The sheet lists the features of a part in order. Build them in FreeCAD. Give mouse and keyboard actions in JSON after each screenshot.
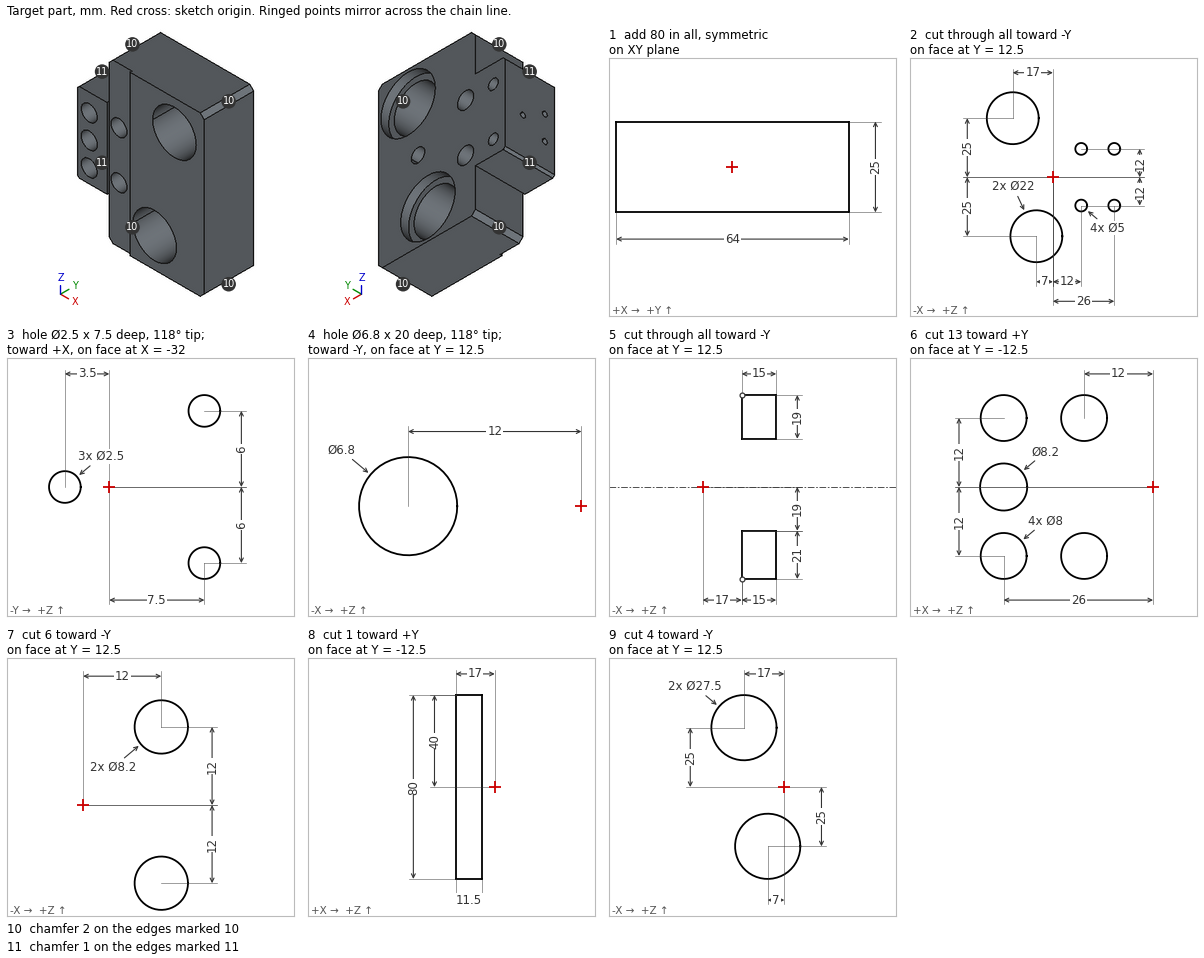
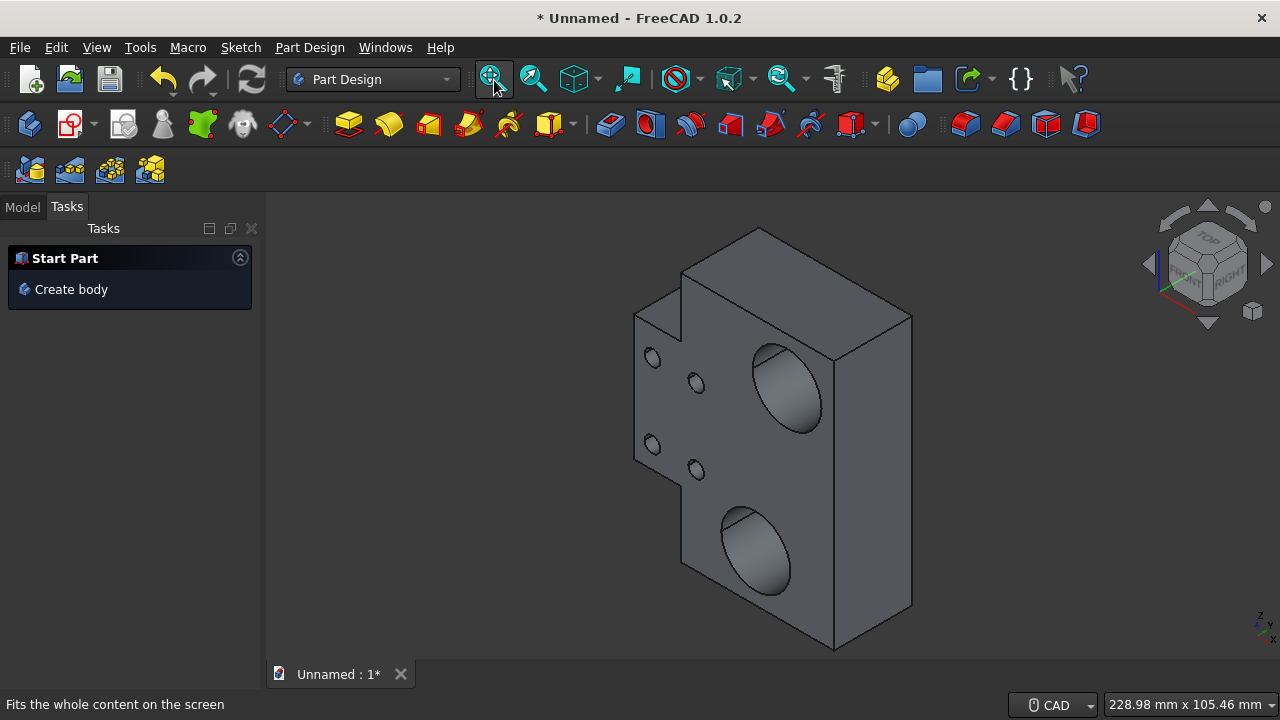
{"action": "left_click", "coordinate": [734, 447]}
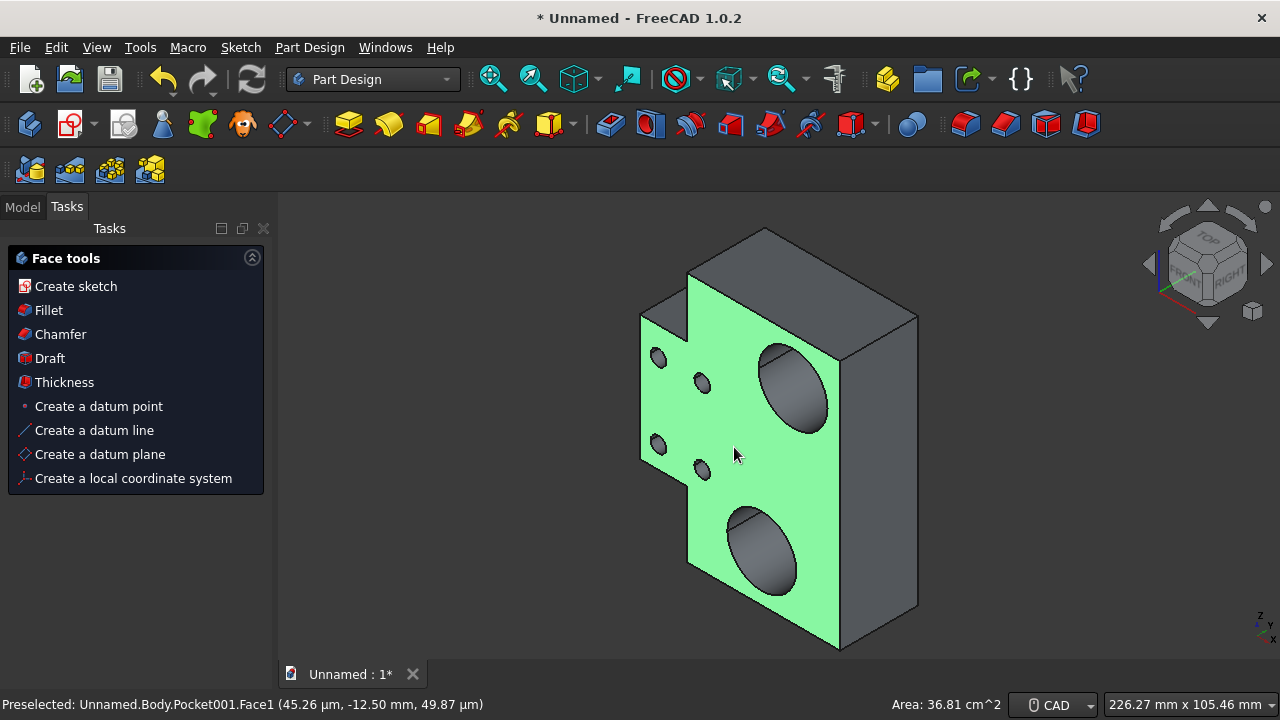
{"action": "left_click", "coordinate": [70, 124]}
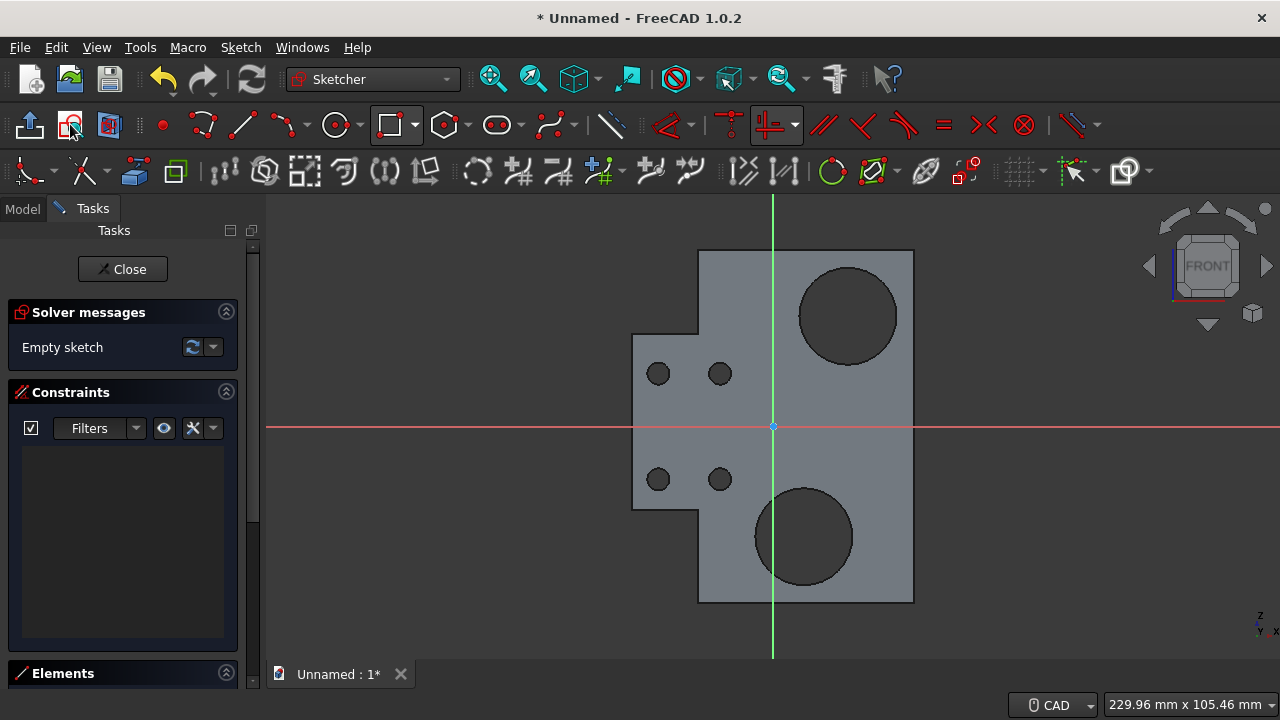
{"action": "scroll", "coordinate": [708, 426], "scroll_direction": "up", "scroll_amount": 4}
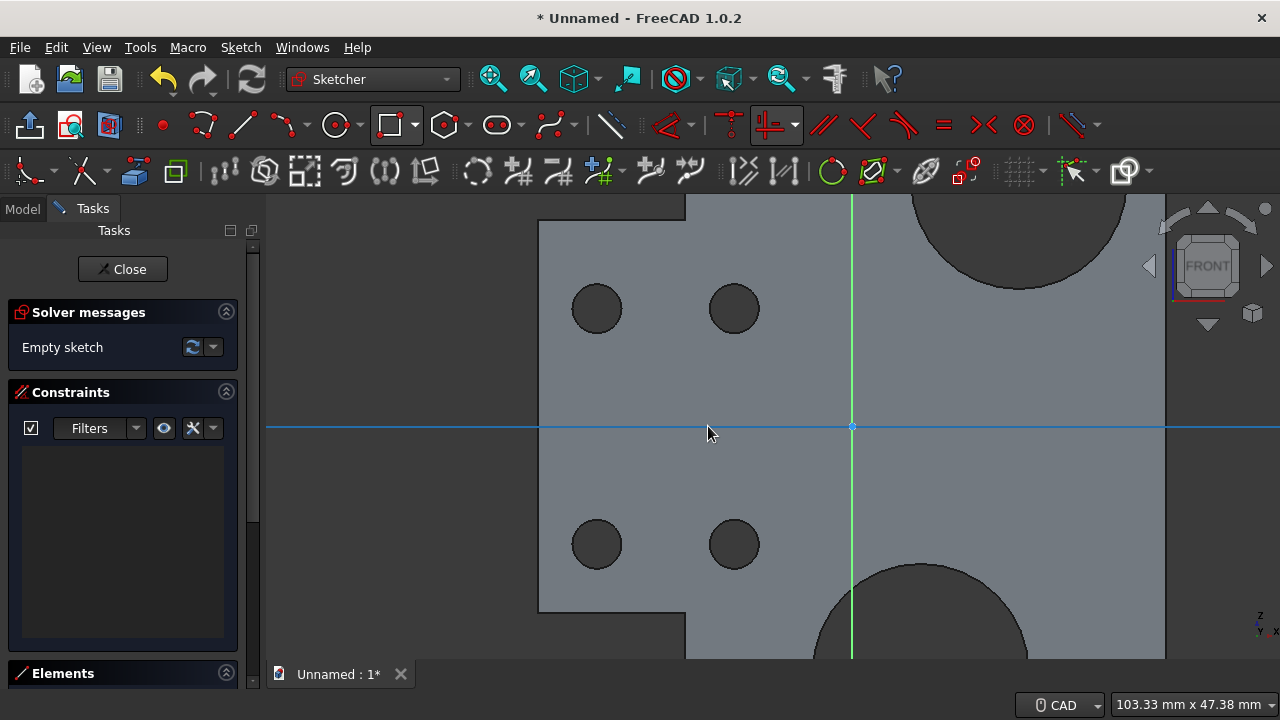
{"action": "left_click", "coordinate": [336, 126]}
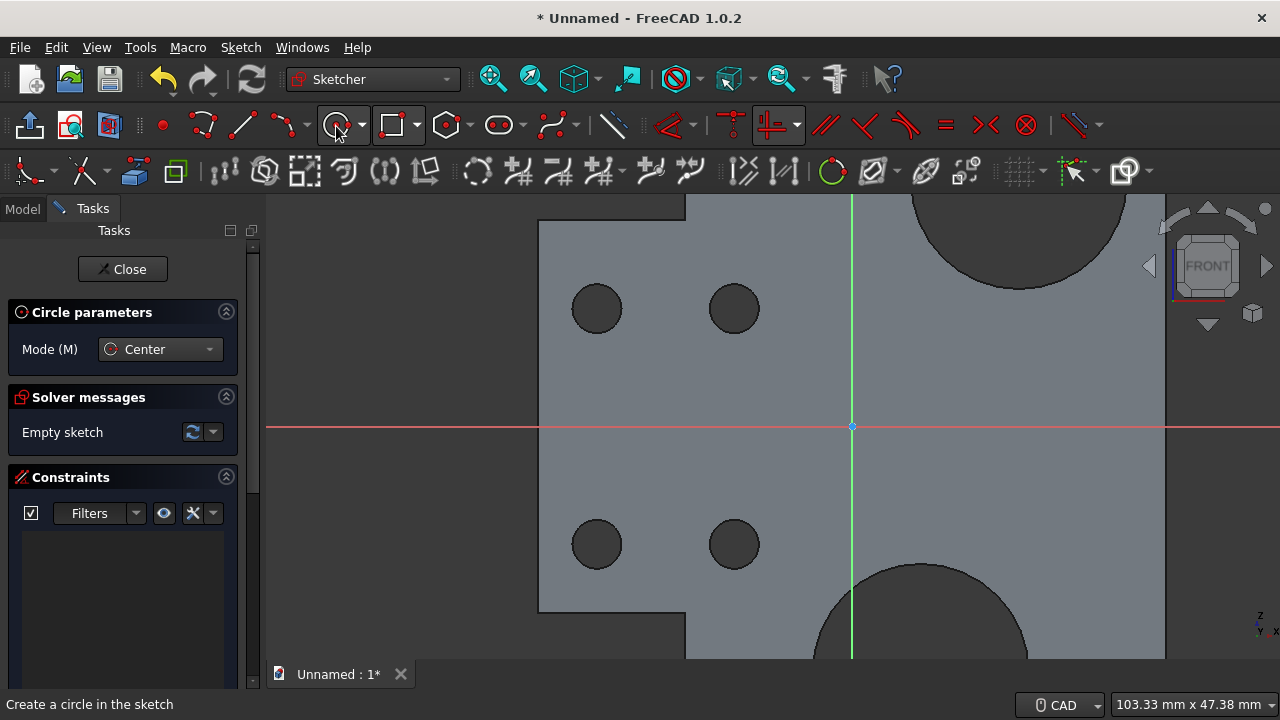
{"action": "left_click", "coordinate": [597, 544]}
{"action": "left_click", "coordinate": [625, 517]}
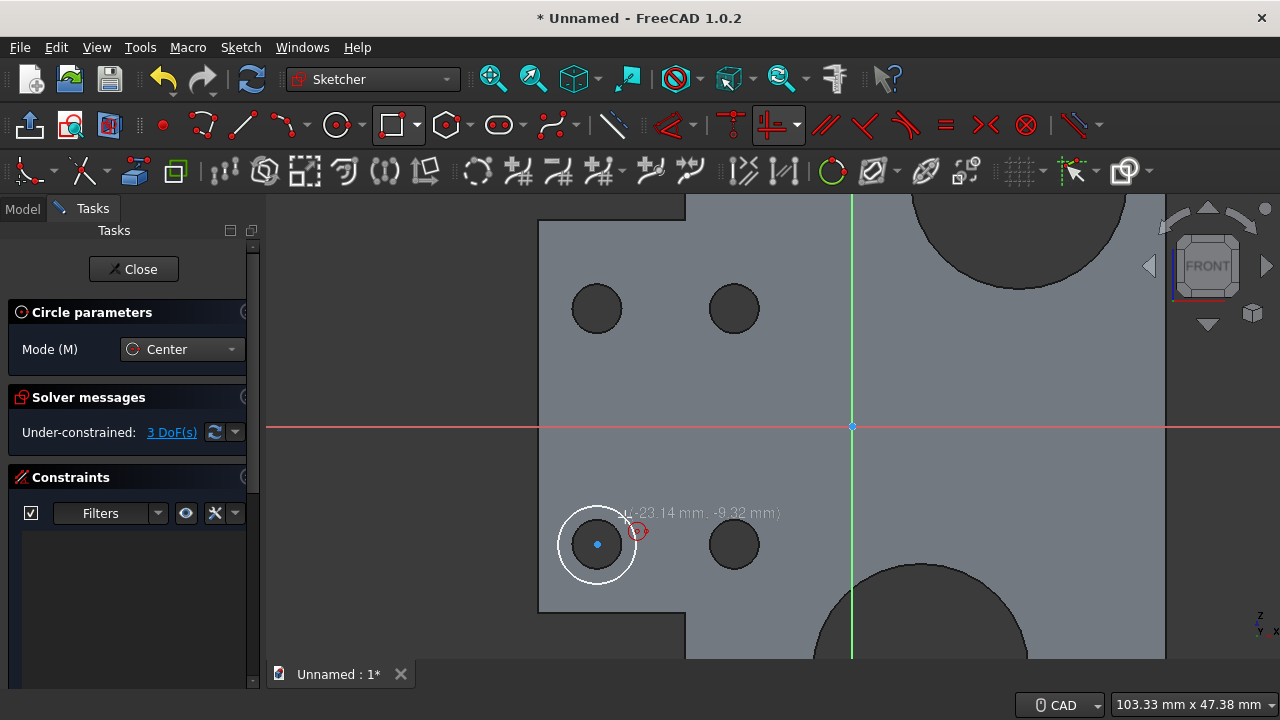
{"action": "left_click", "coordinate": [597, 309]}
{"action": "left_click", "coordinate": [625, 281]}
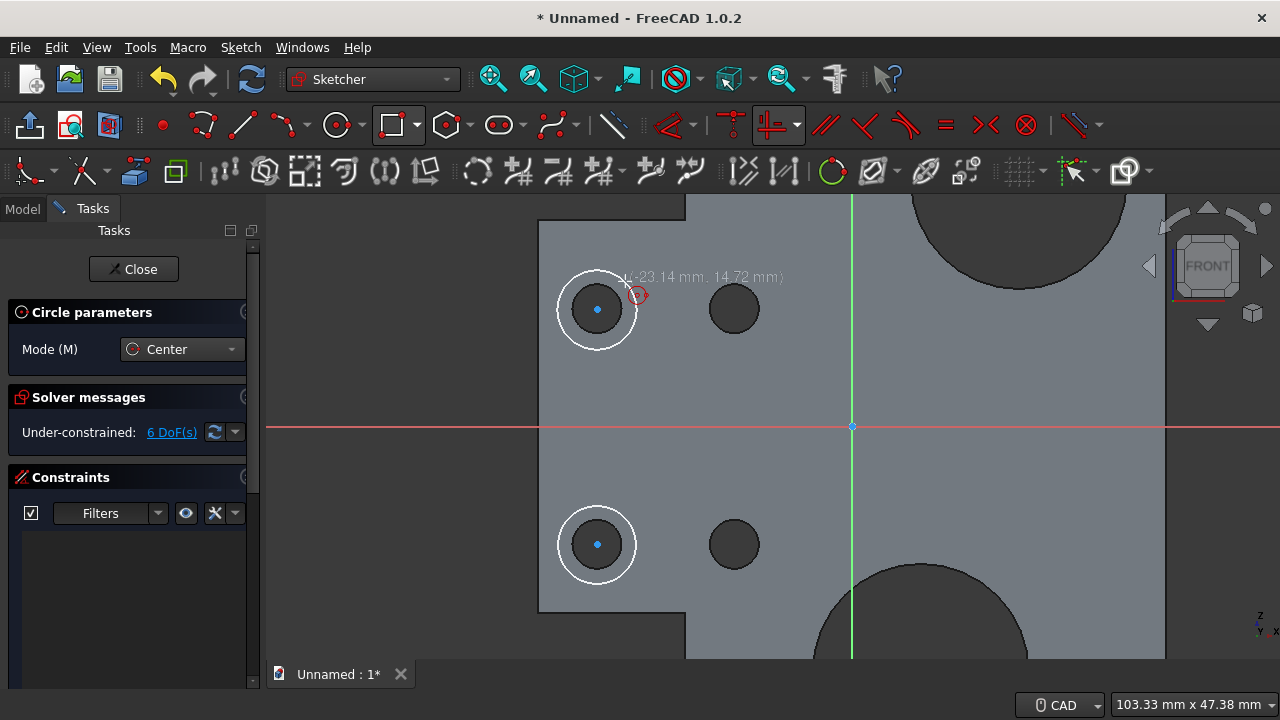
{"action": "left_click", "coordinate": [734, 309]}
{"action": "left_click", "coordinate": [762, 281]}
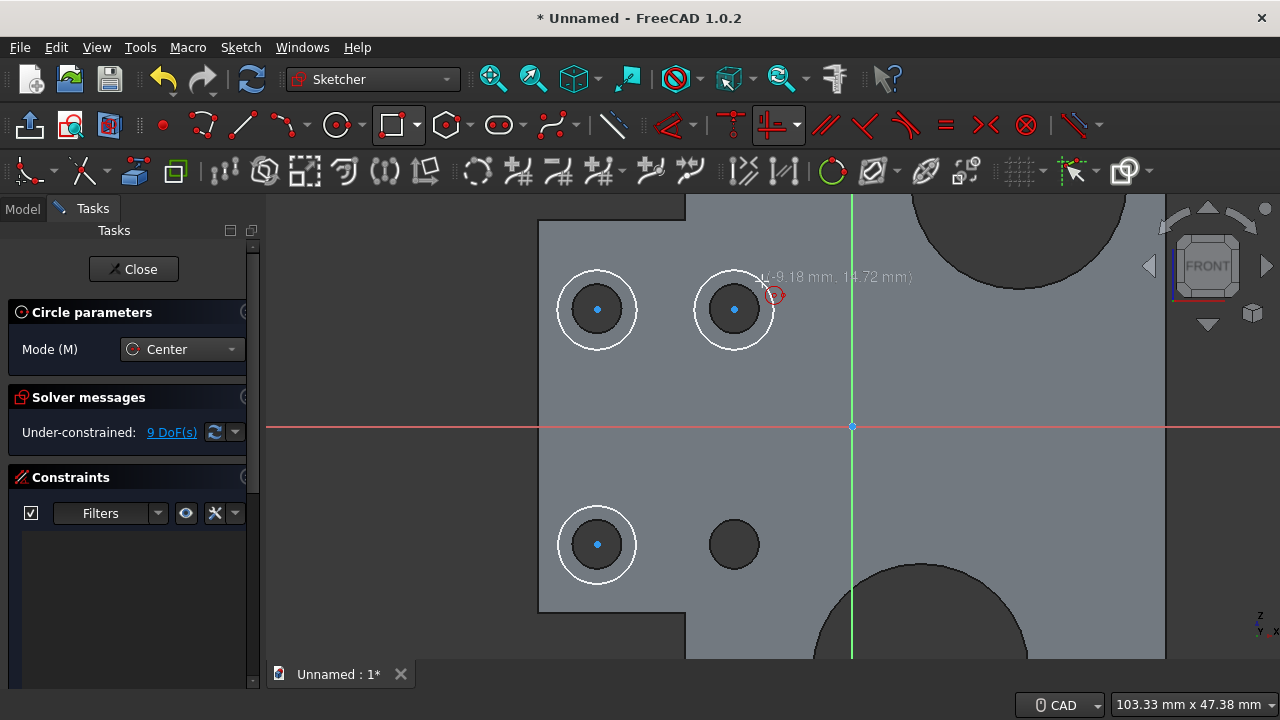
{"action": "left_click", "coordinate": [734, 544]}
{"action": "left_click", "coordinate": [762, 517]}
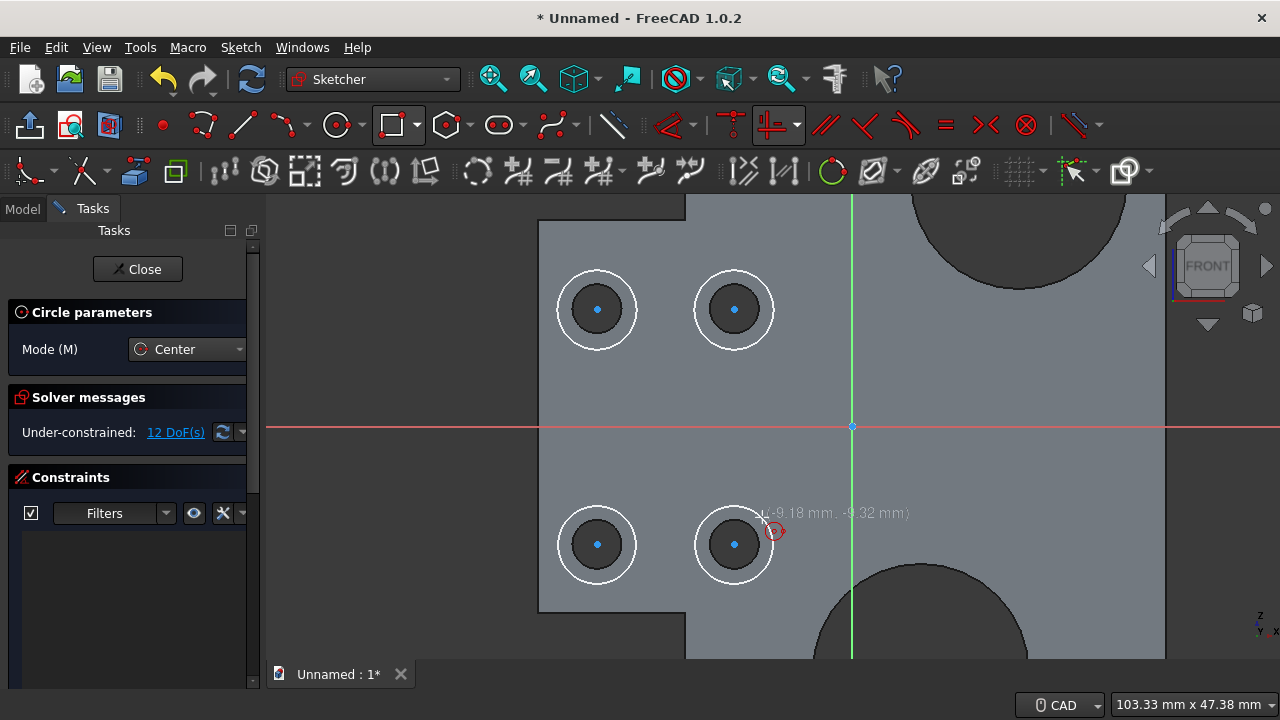
{"action": "left_click", "coordinate": [597, 426]}
{"action": "left_click", "coordinate": [625, 398]}
{"action": "key", "text": "Escape"}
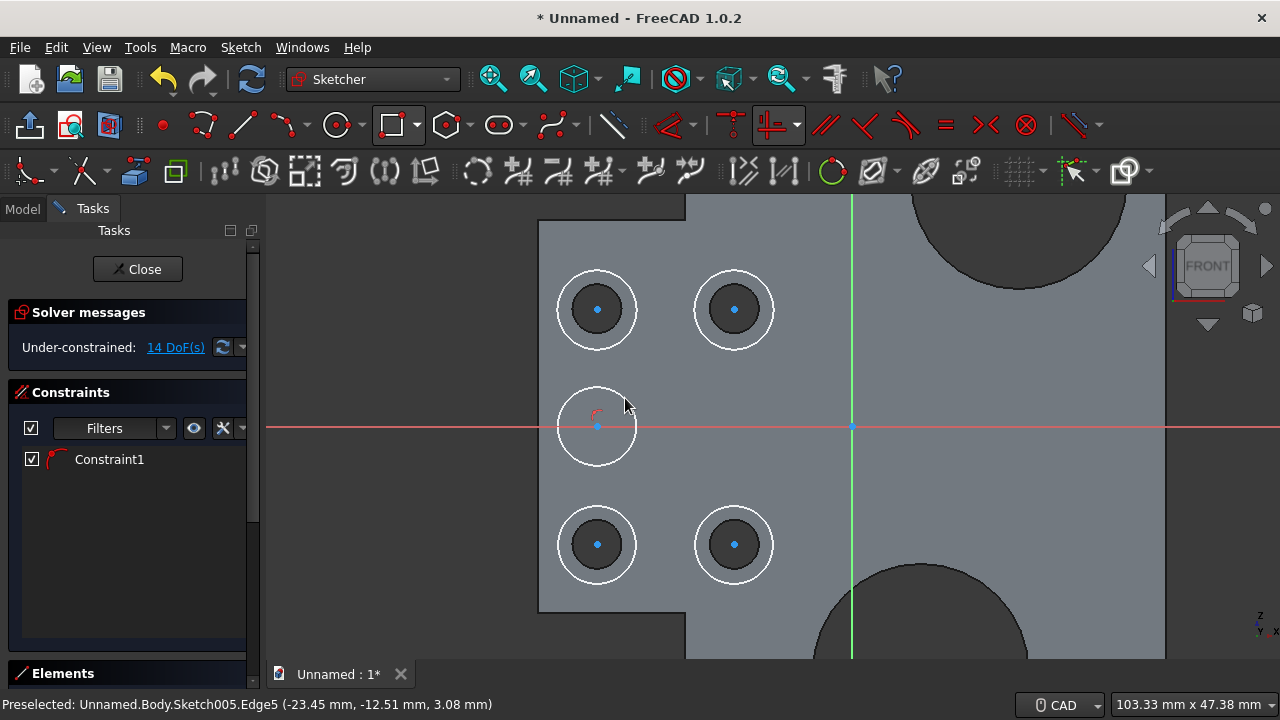
{"action": "left_click", "coordinate": [624, 517]}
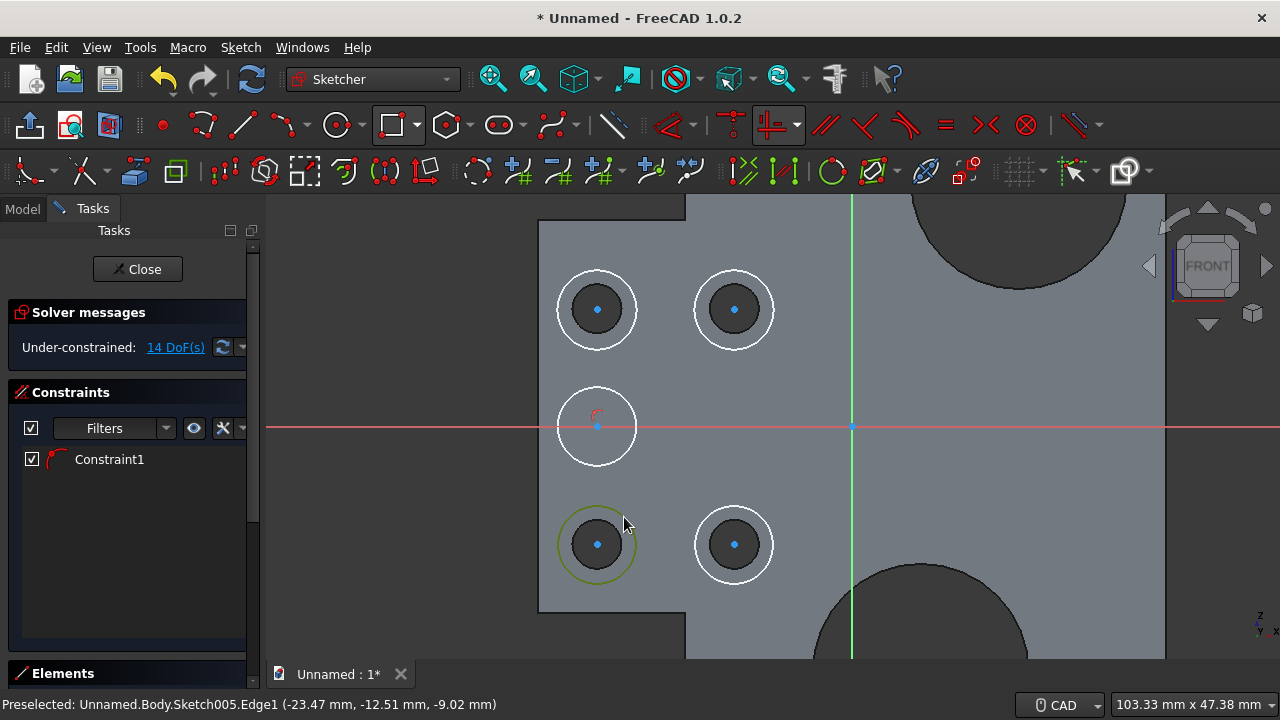
{"action": "left_click", "coordinate": [625, 282]}